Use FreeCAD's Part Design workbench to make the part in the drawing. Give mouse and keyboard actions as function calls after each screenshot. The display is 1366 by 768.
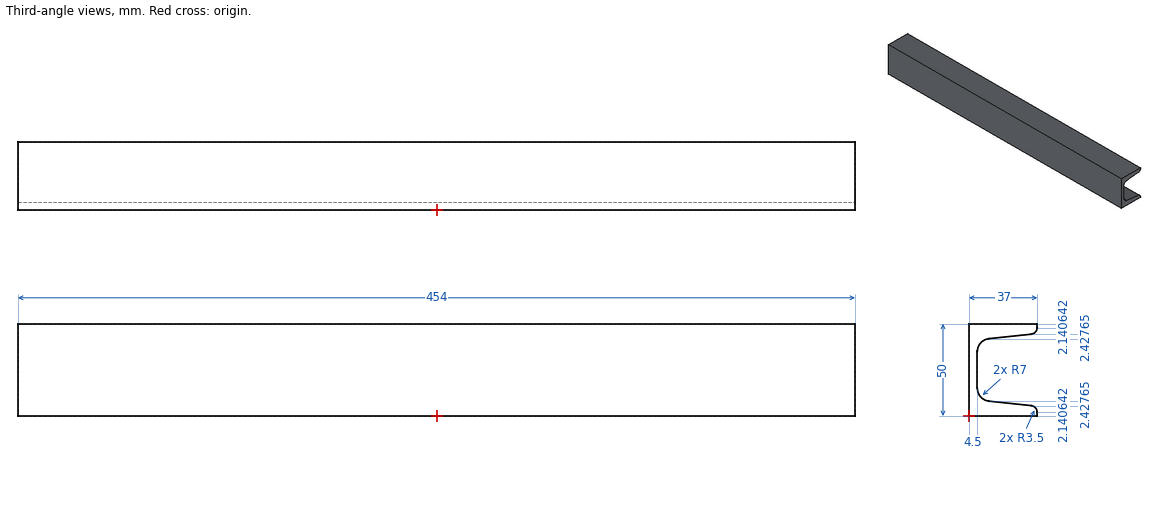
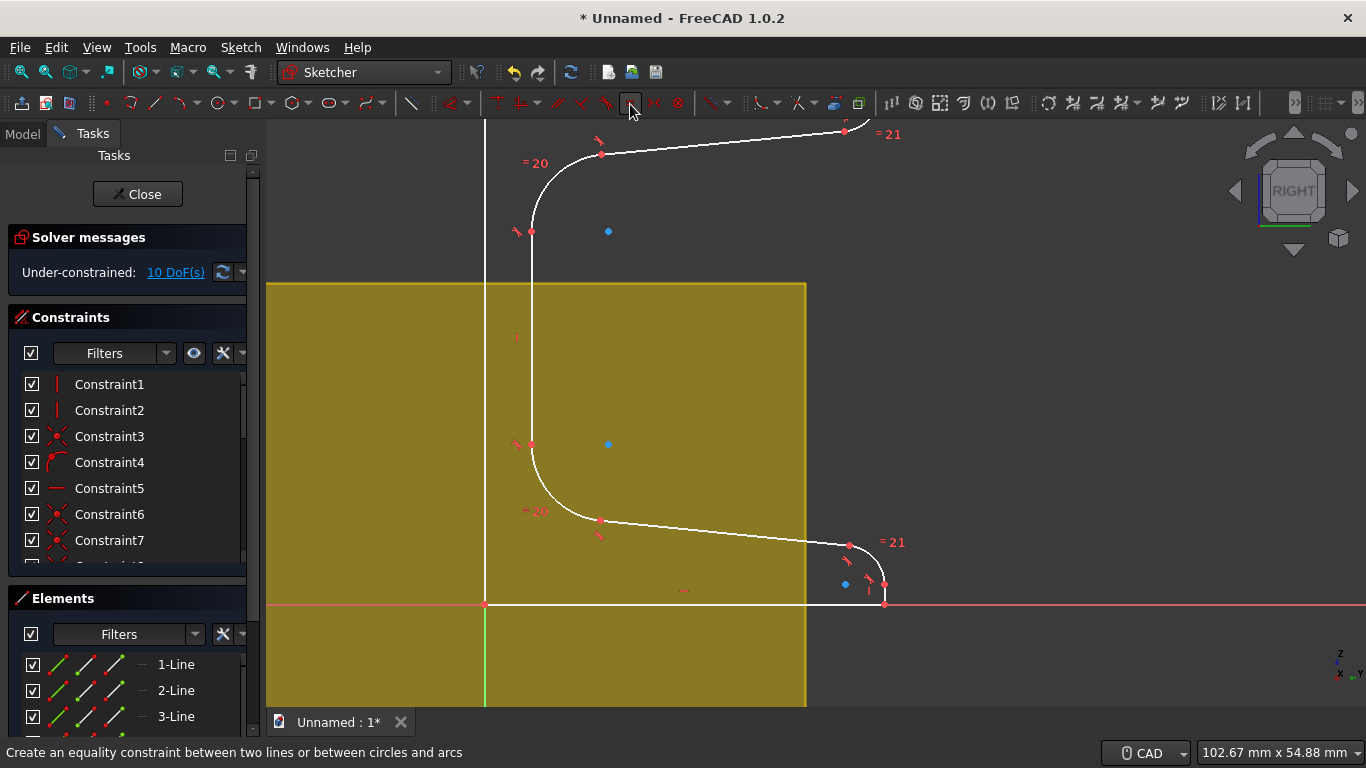
click(539, 477)
click(510, 491)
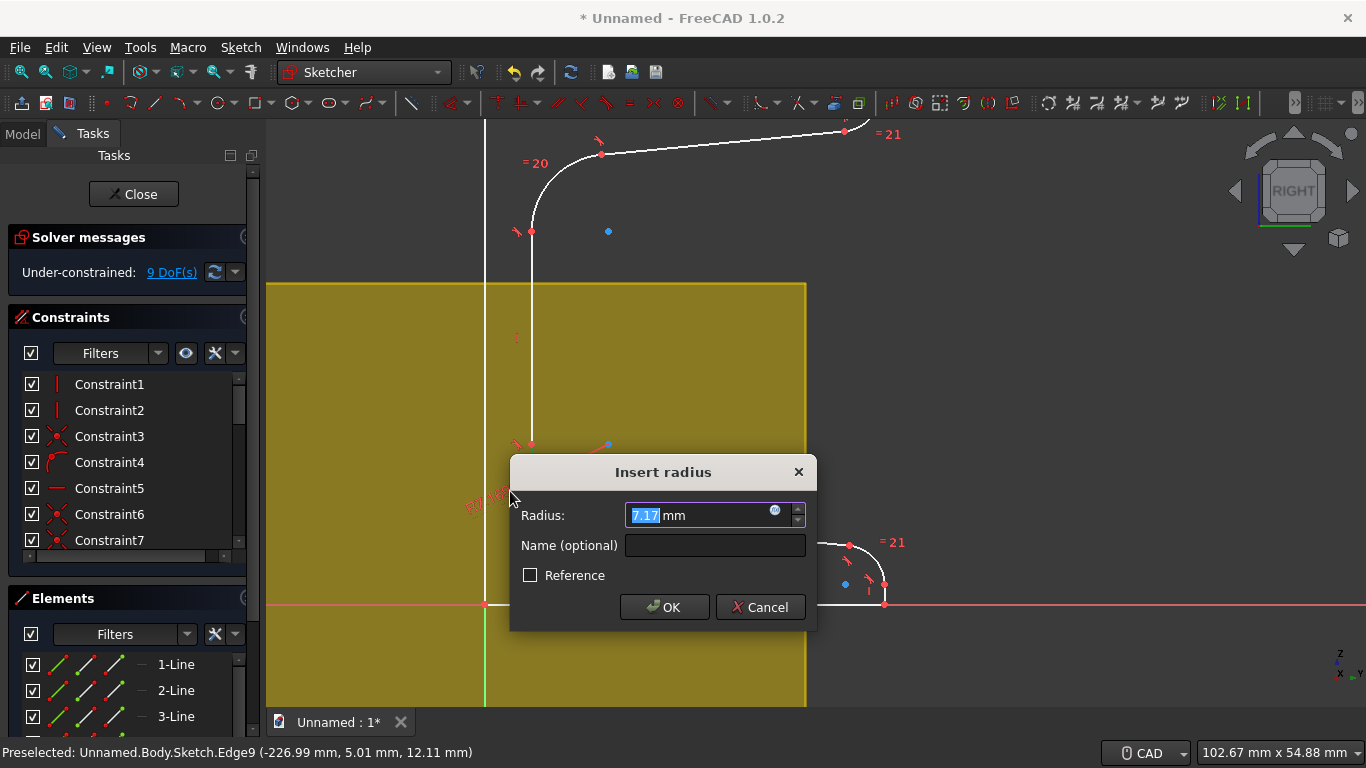
text(7)
key(Return)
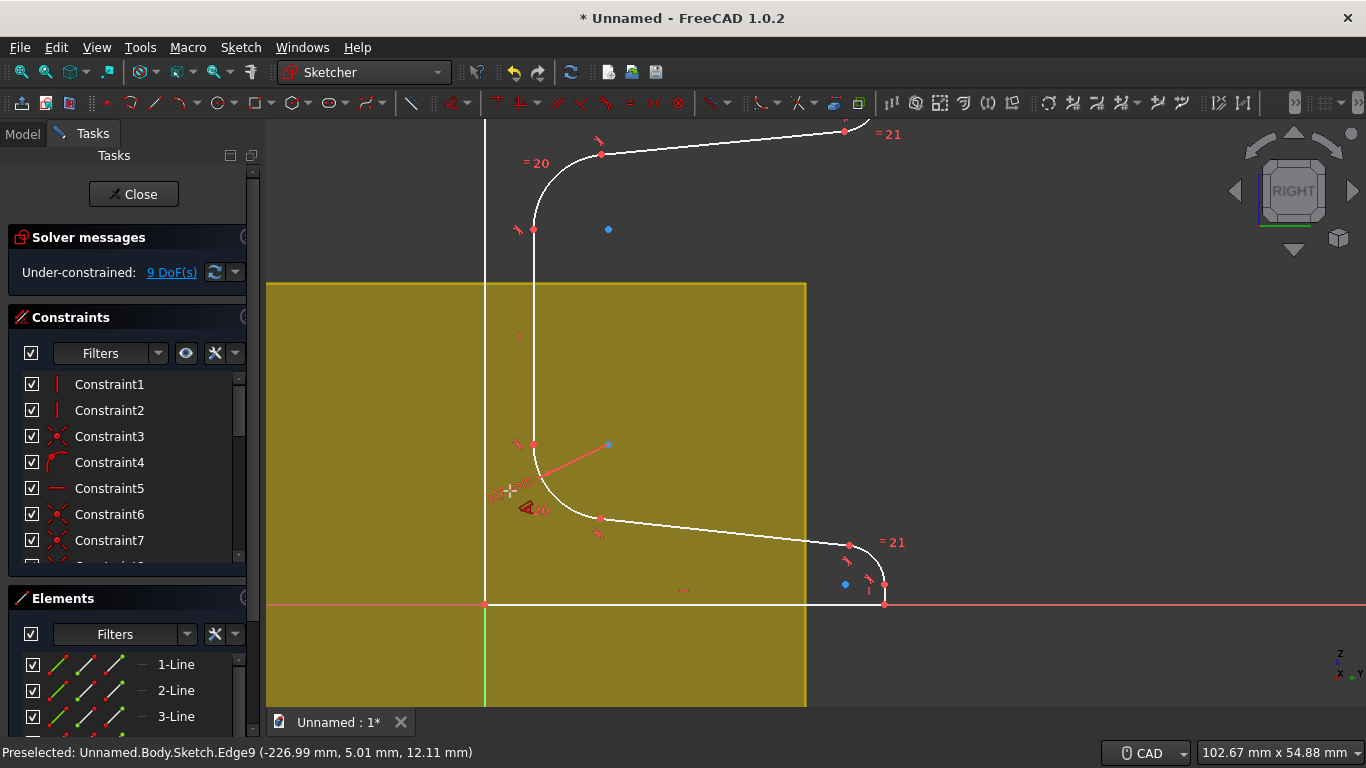
scroll(879, 568, down, 2)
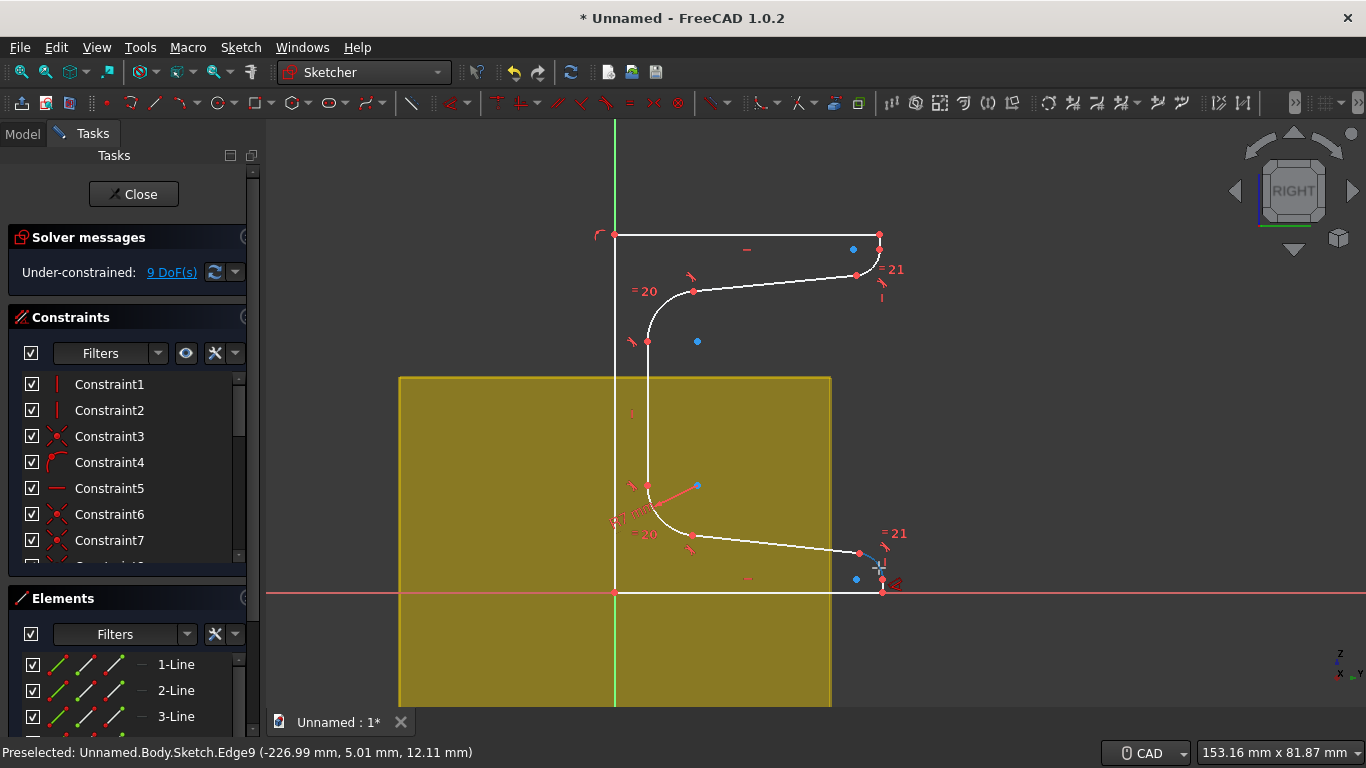
scroll(867, 272, up, 3)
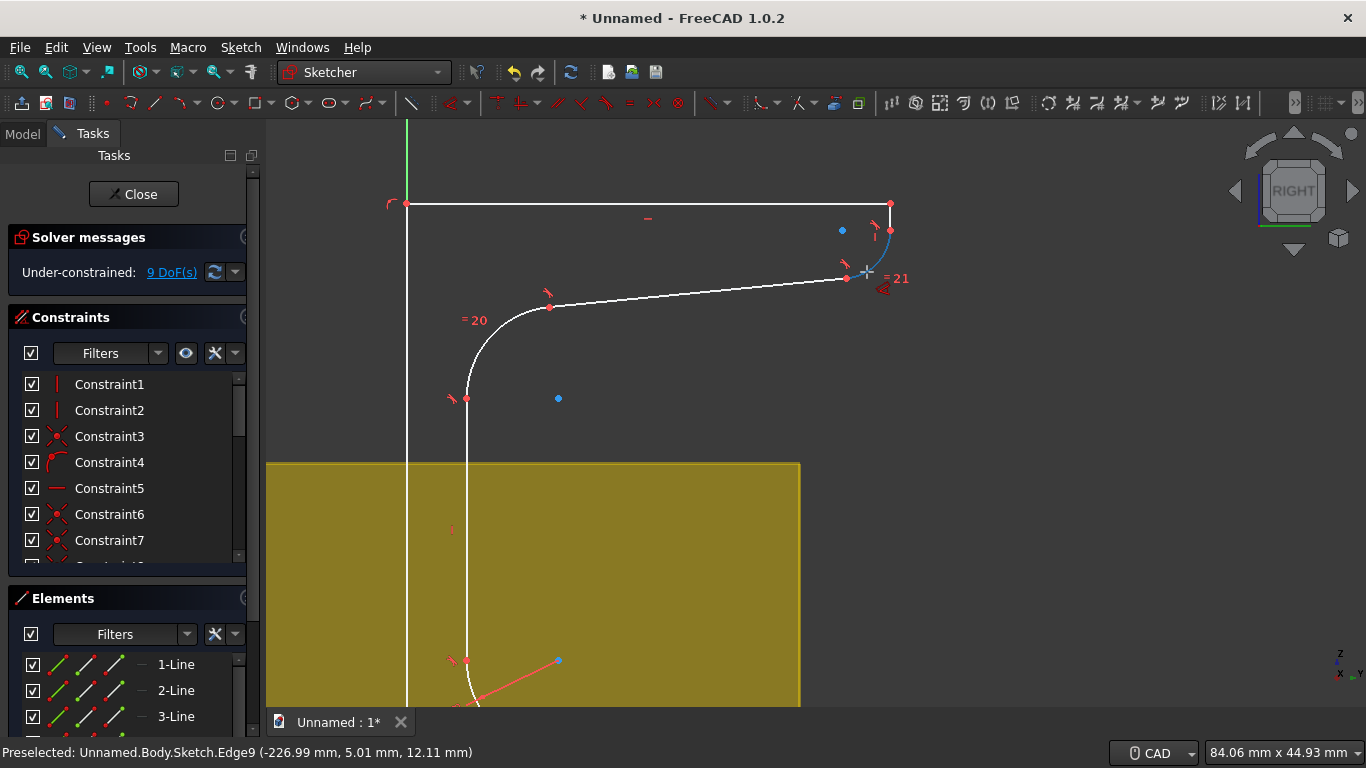
click(867, 272)
click(883, 299)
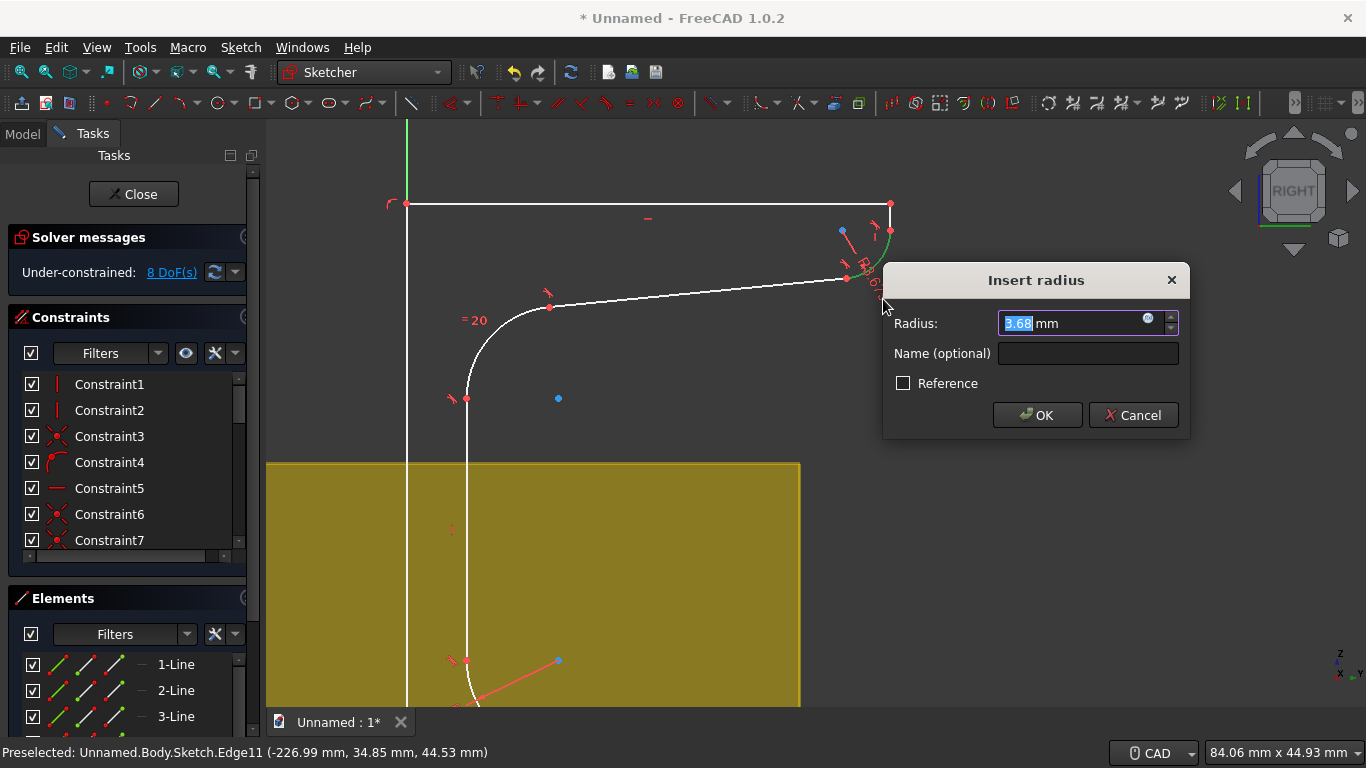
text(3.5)
key(Return)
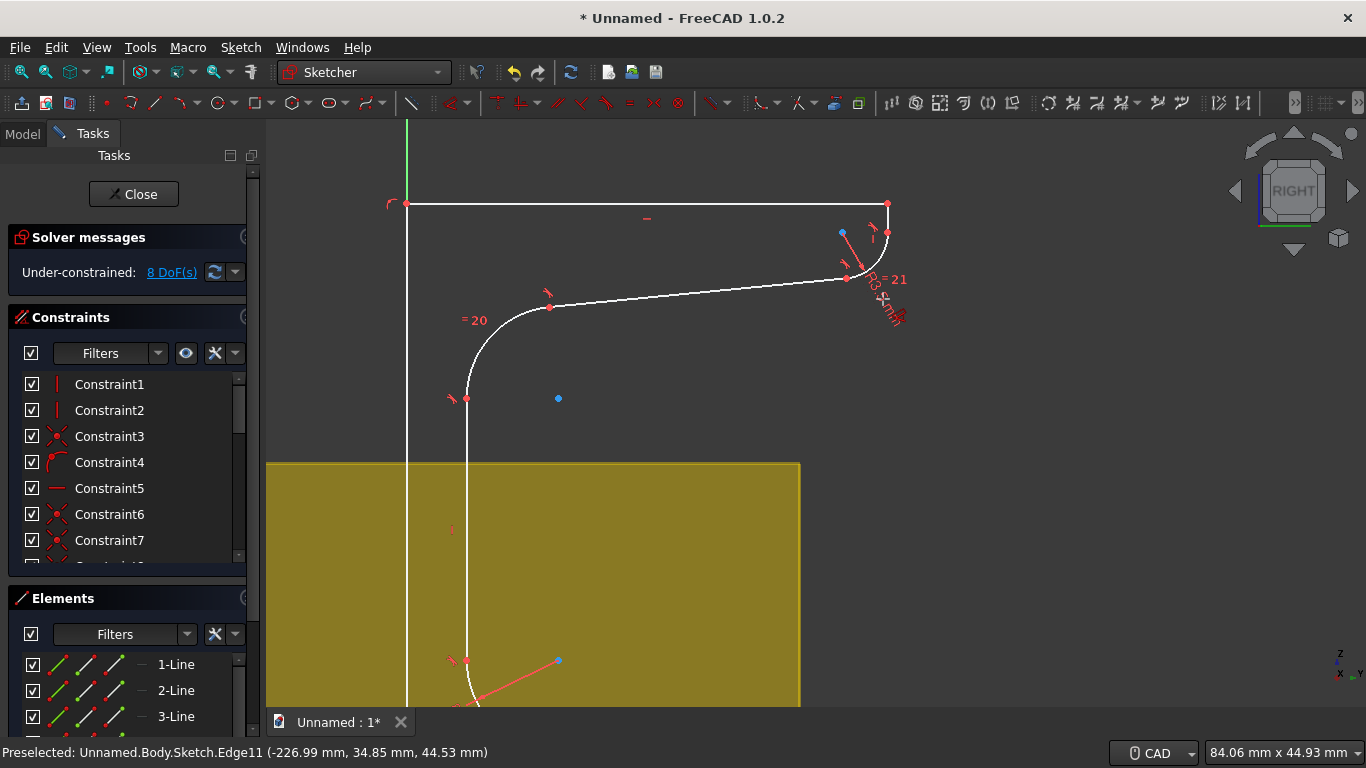
click(744, 204)
click(647, 170)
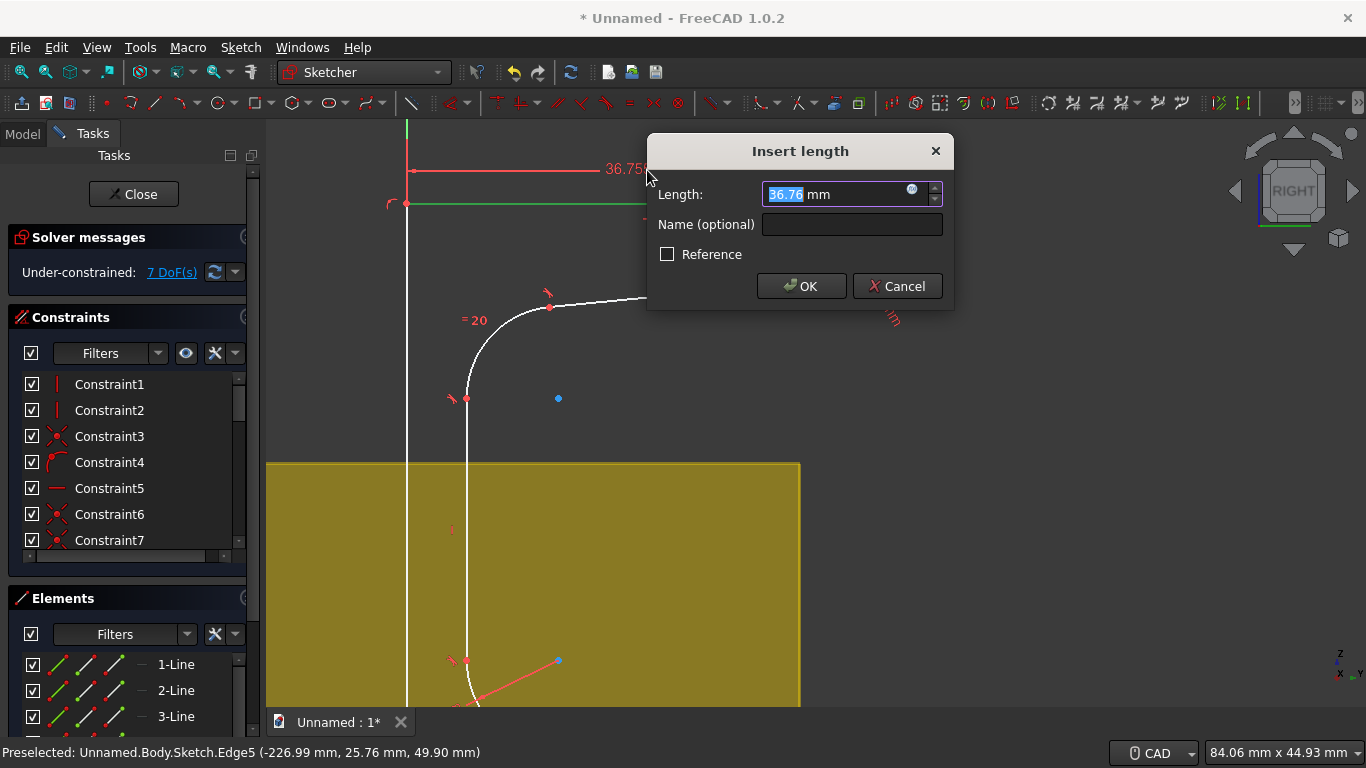
text(37)
key(Return)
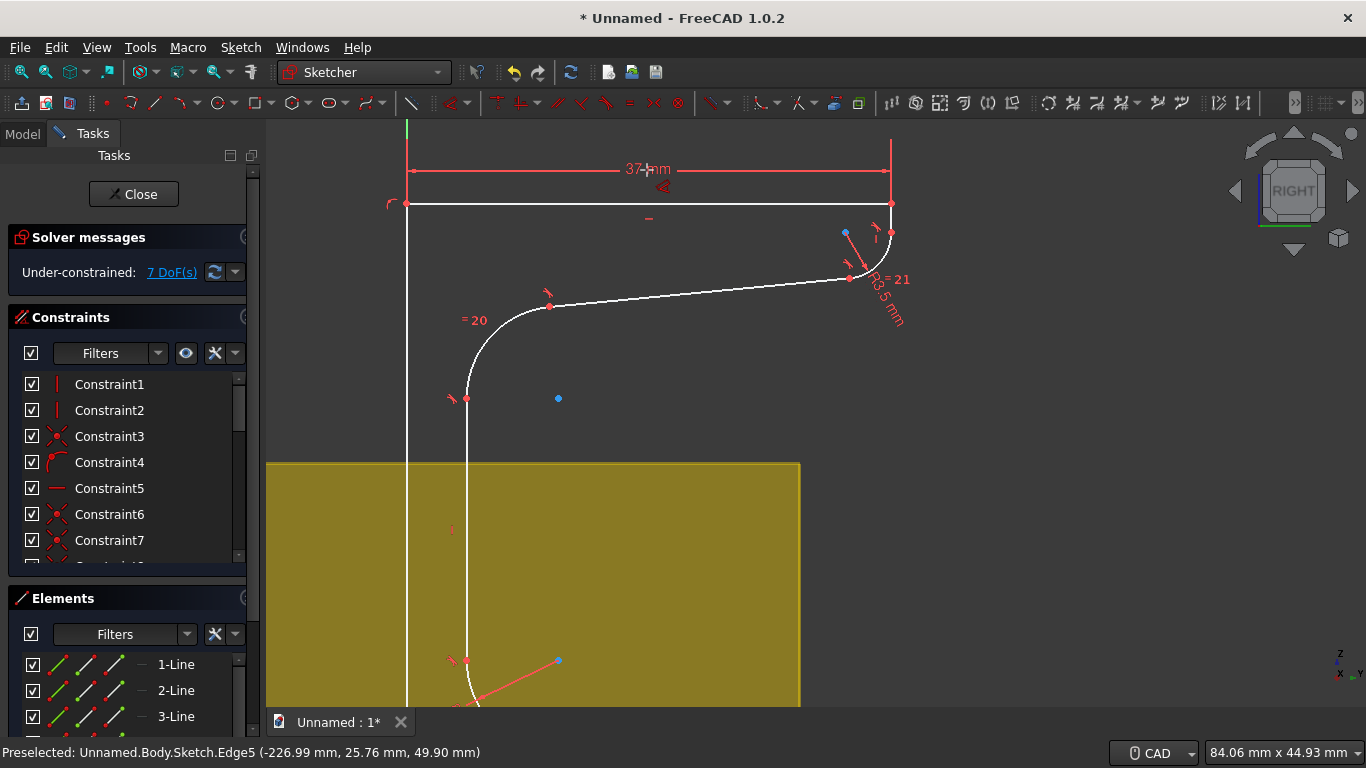
click(407, 399)
click(373, 441)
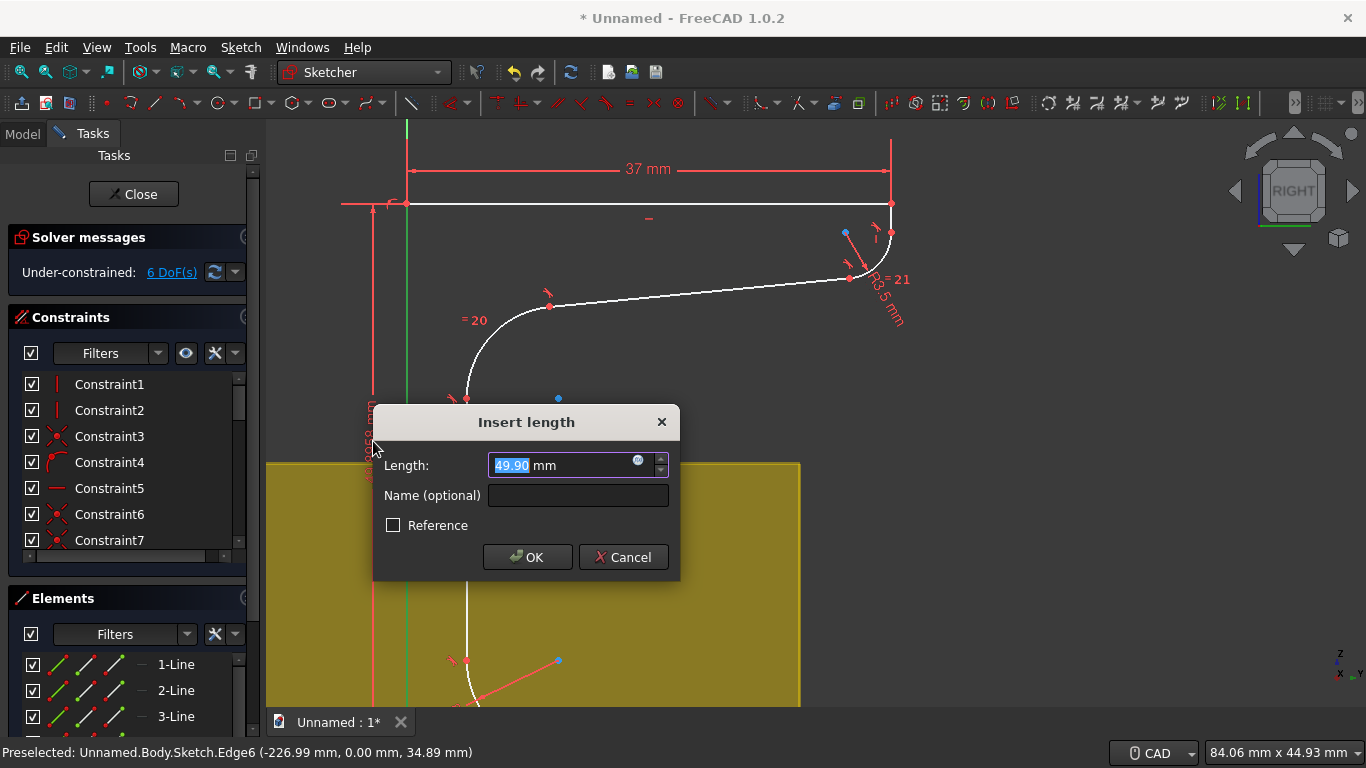
text(50)
key(Return)